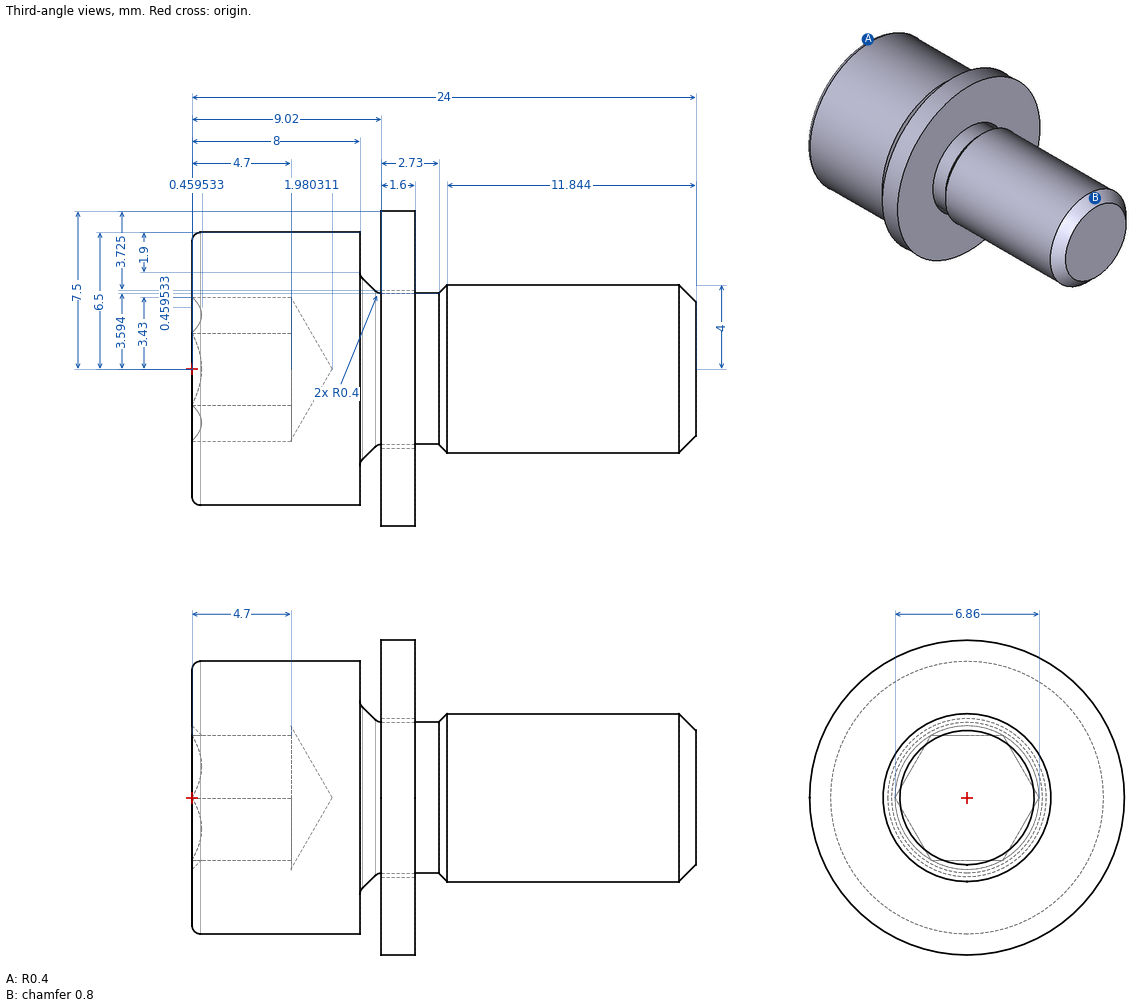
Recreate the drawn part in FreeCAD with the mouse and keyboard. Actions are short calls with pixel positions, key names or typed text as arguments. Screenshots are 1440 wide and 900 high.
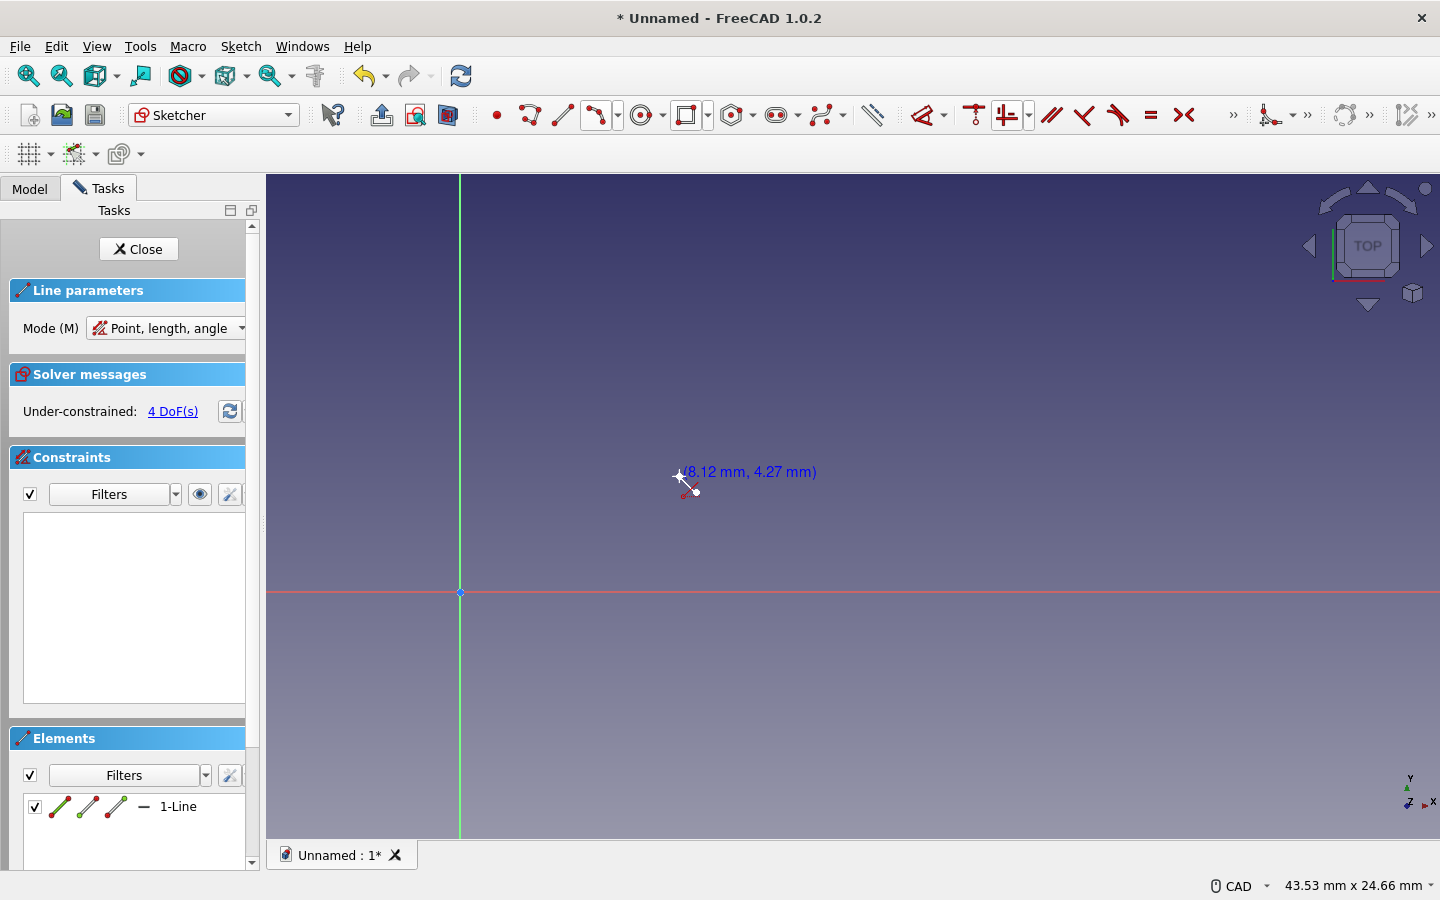
click(530, 116)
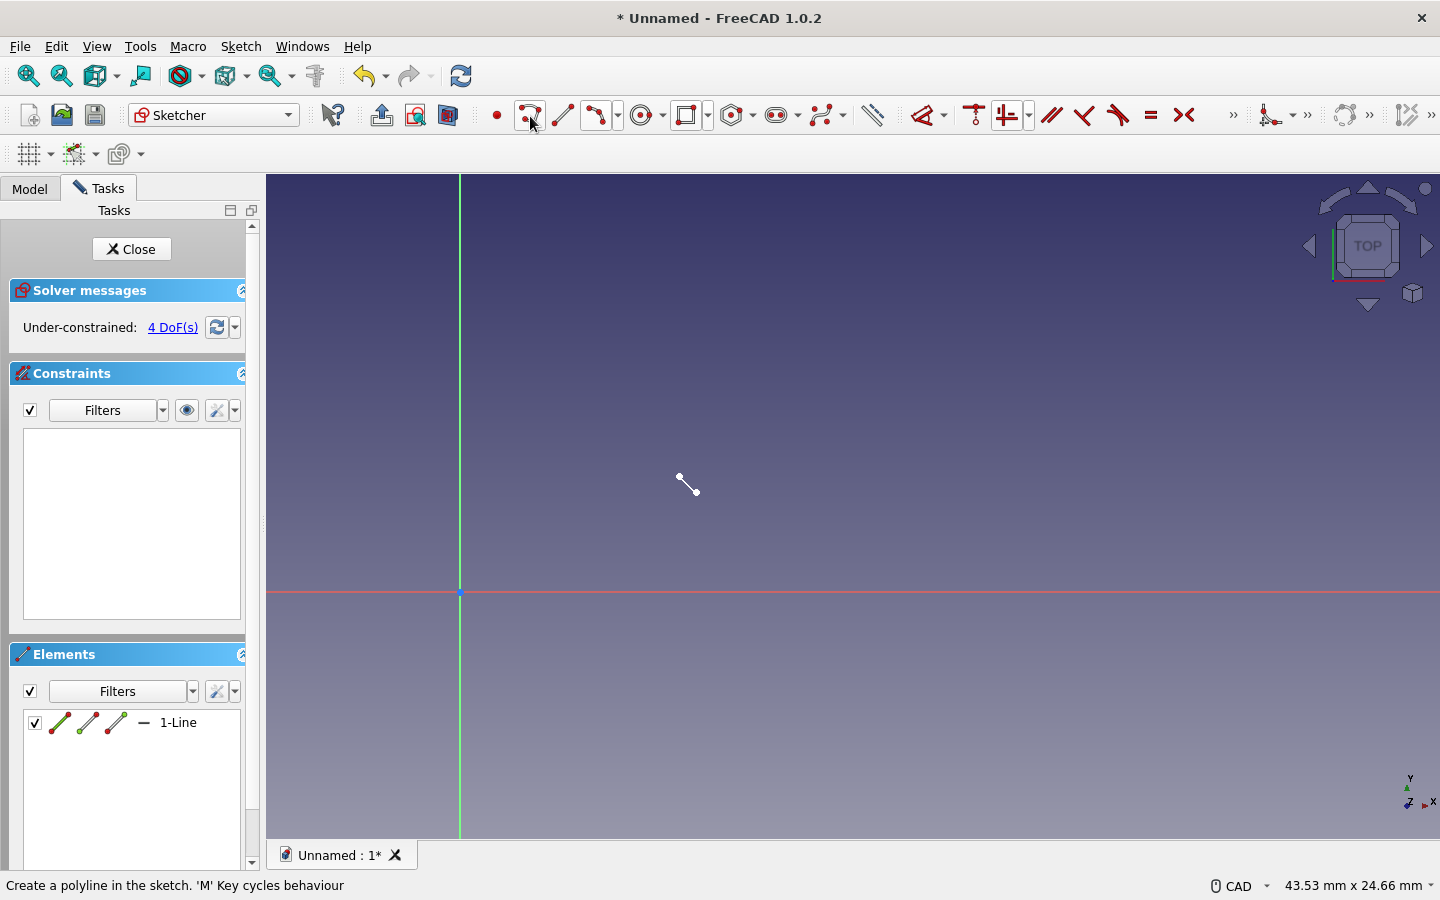
scroll(676, 468, up, 4)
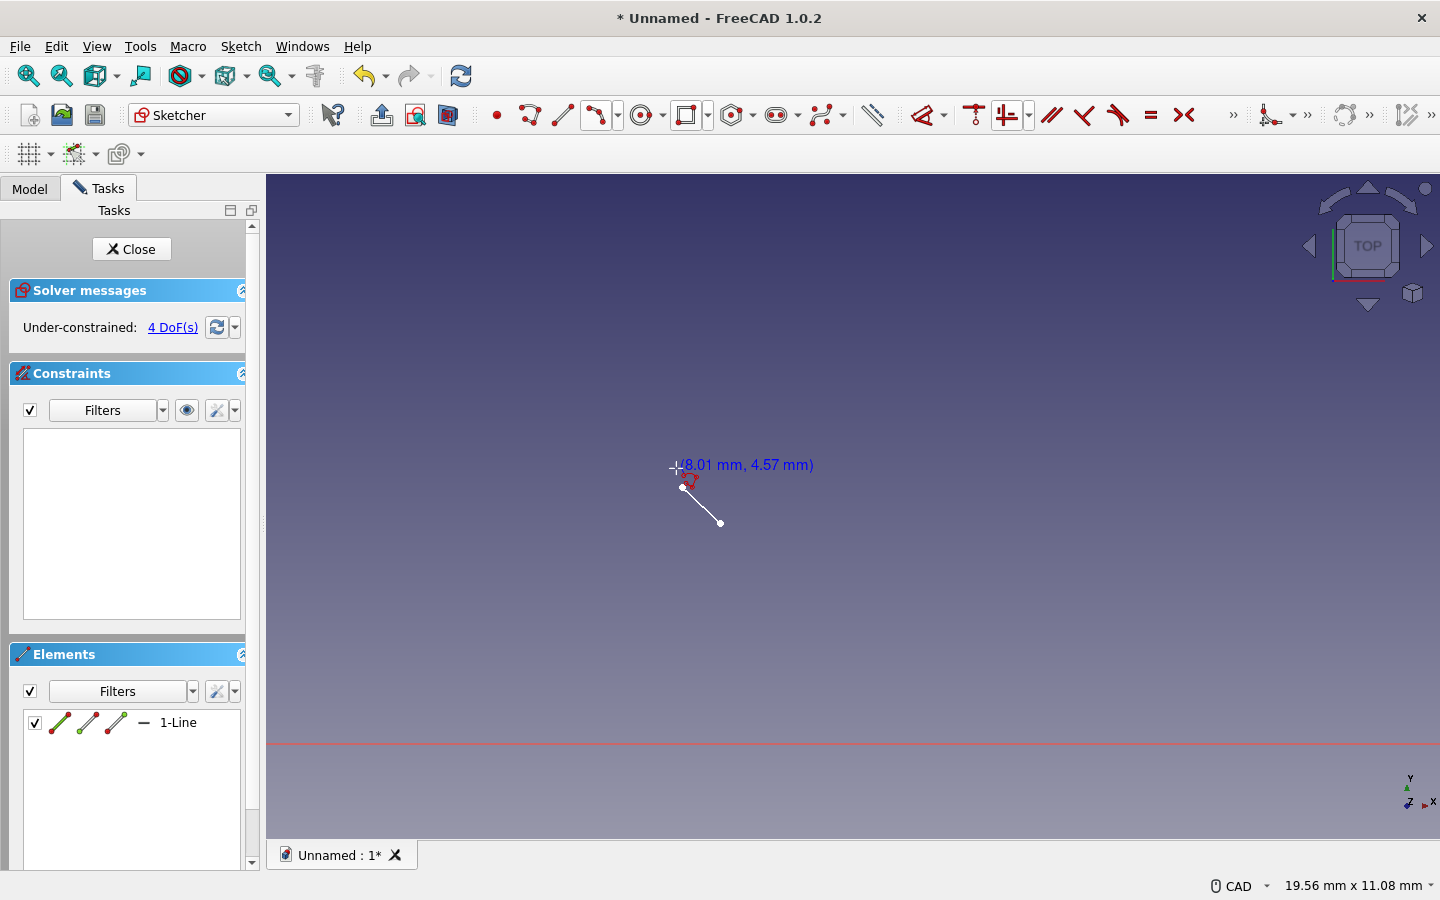
click(675, 468)
click(675, 354)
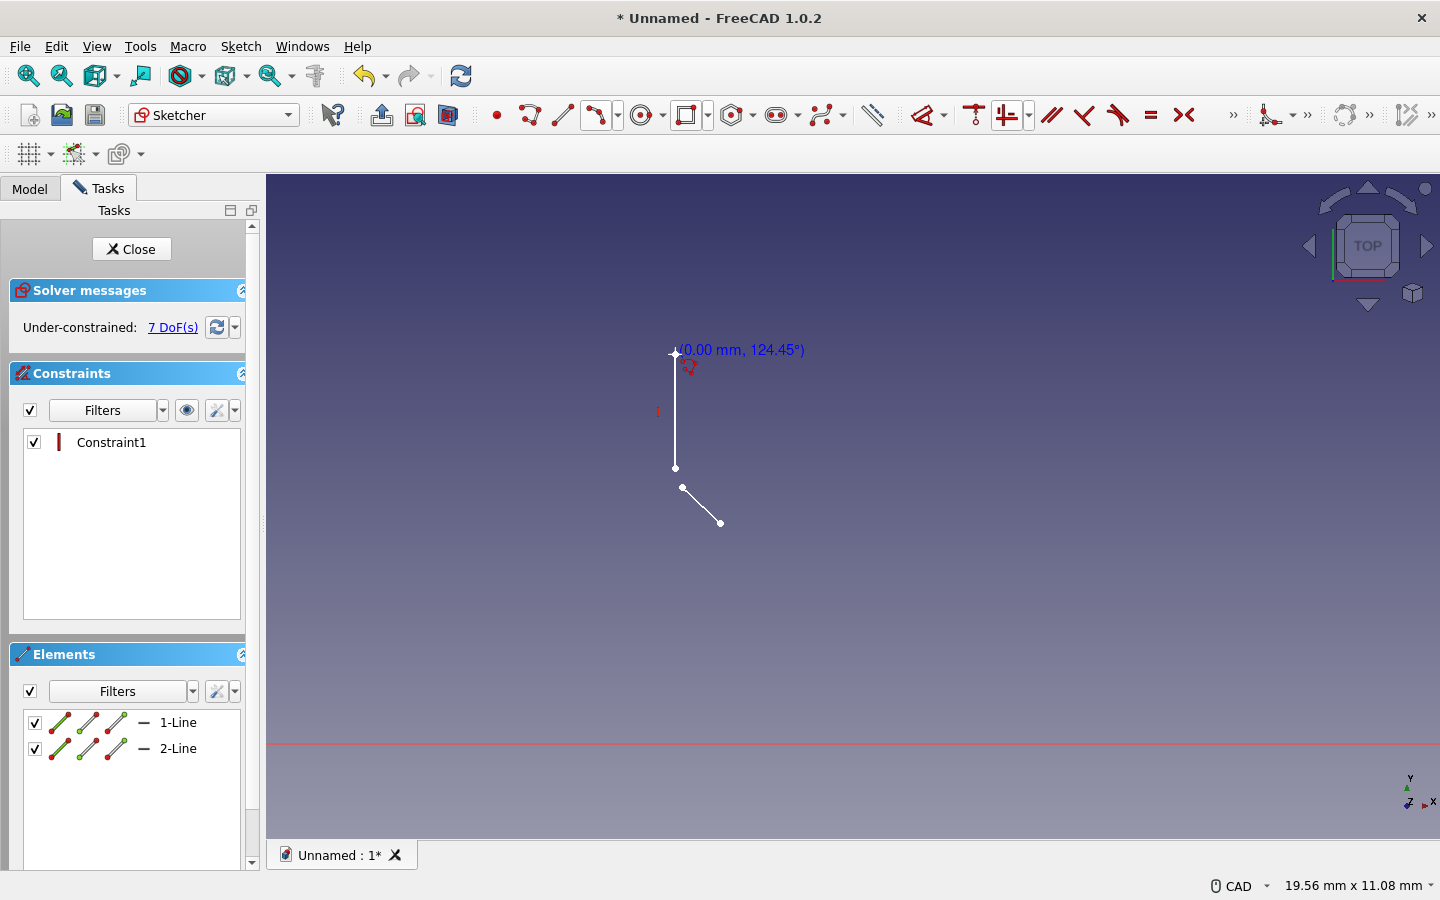
scroll(678, 472, down, 4)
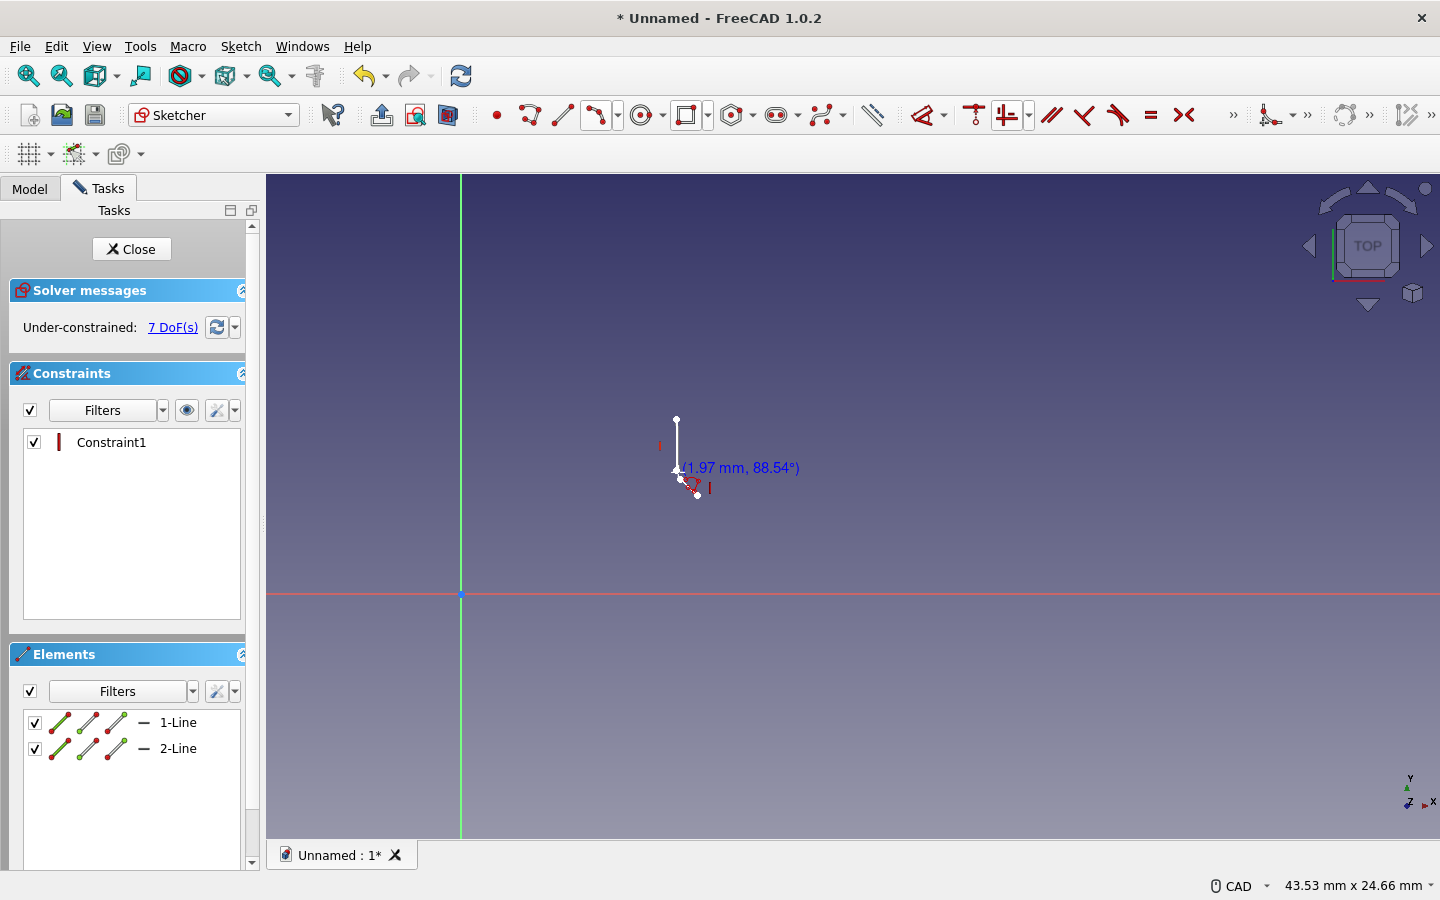
click(461, 419)
click(461, 594)
click(1108, 585)
click(1108, 487)
click(789, 487)
click(778, 497)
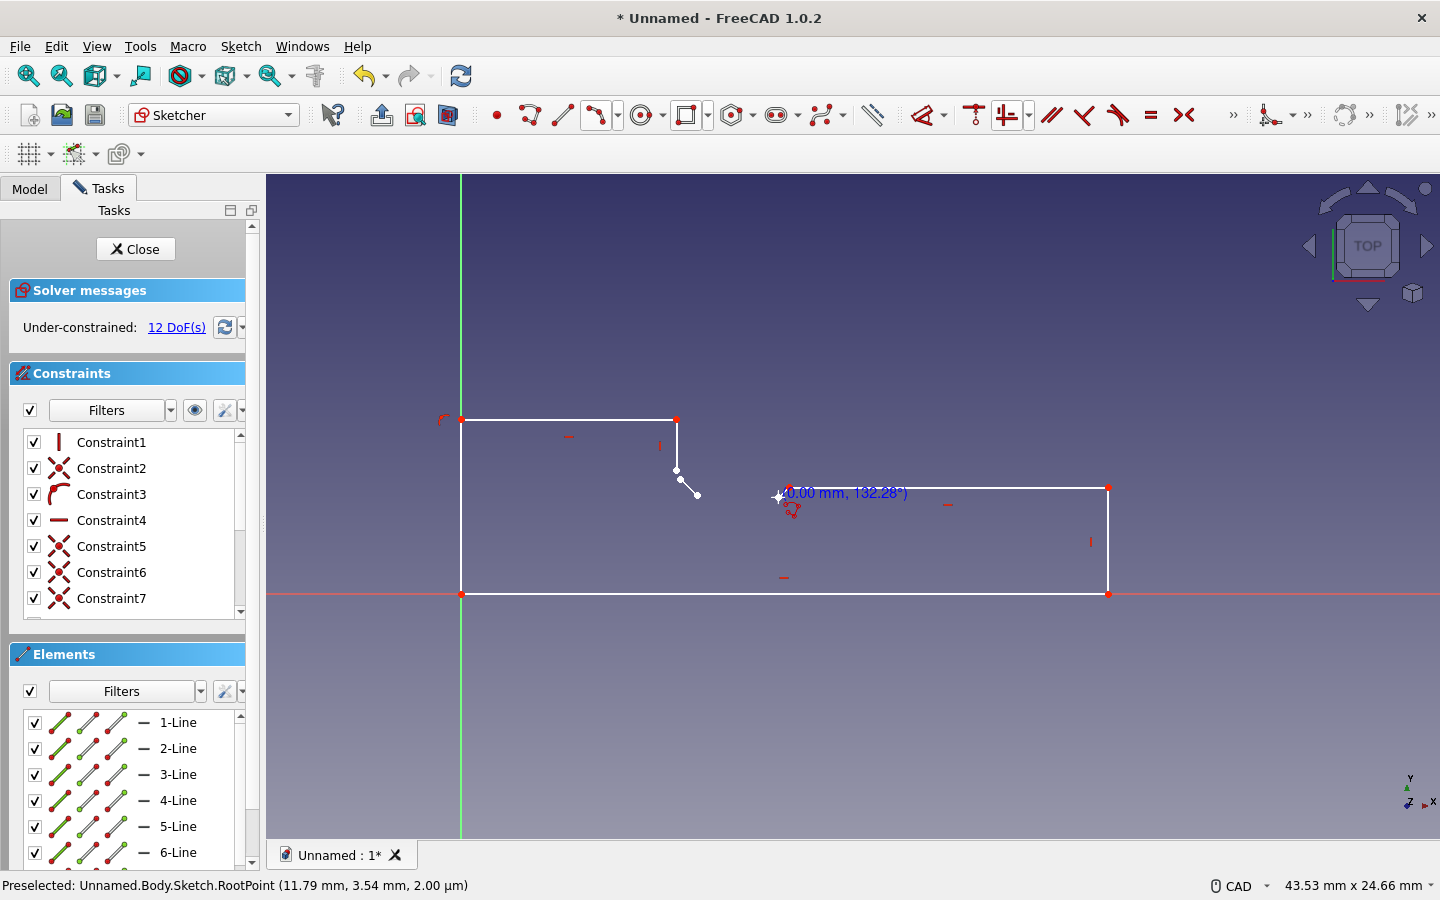
scroll(704, 497, up, 4)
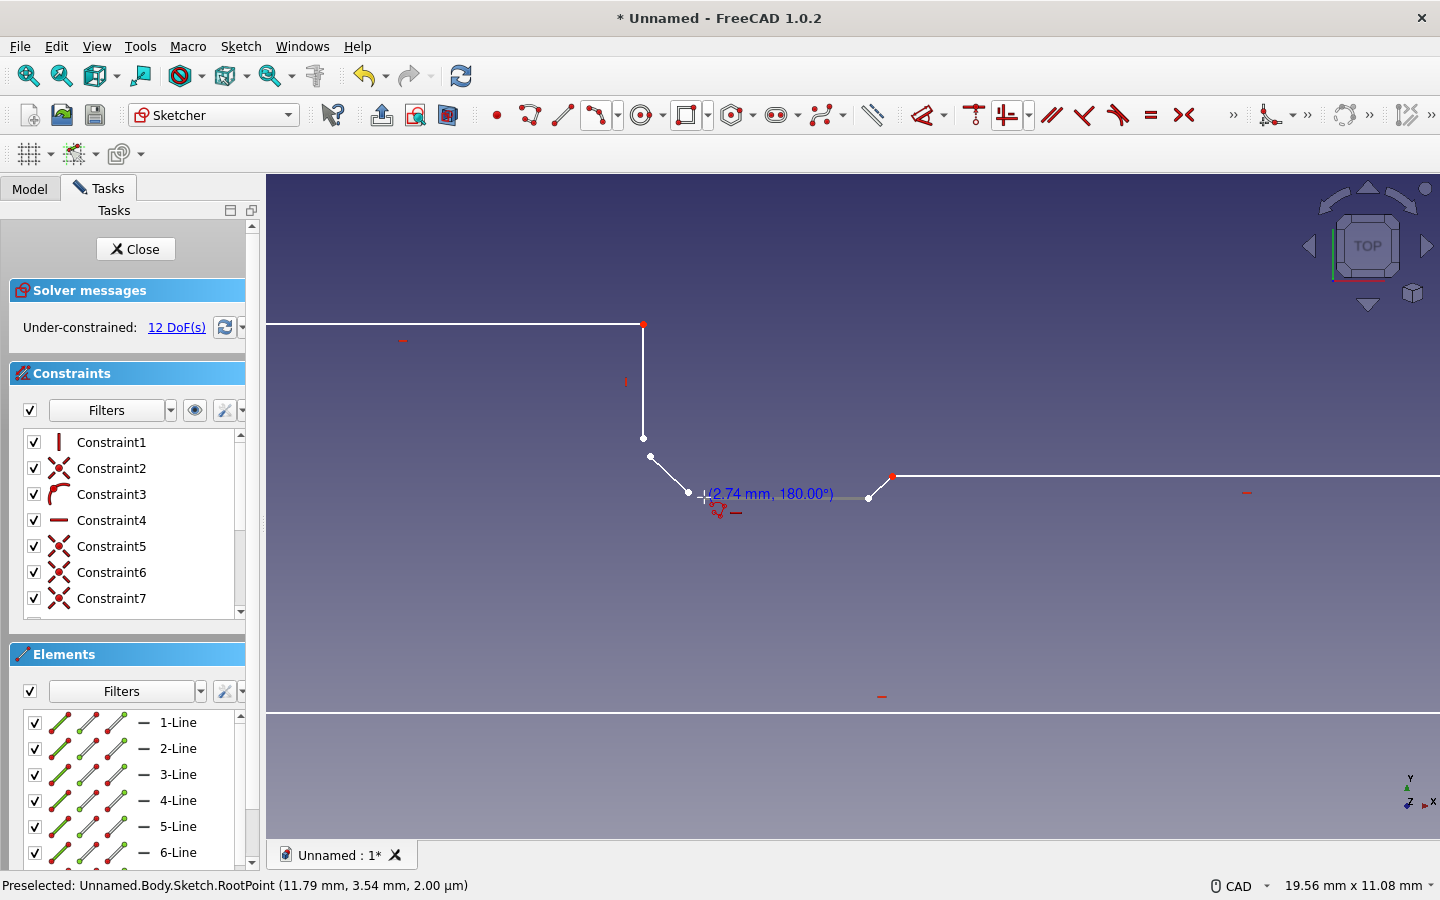
click(704, 496)
right_click(704, 496)